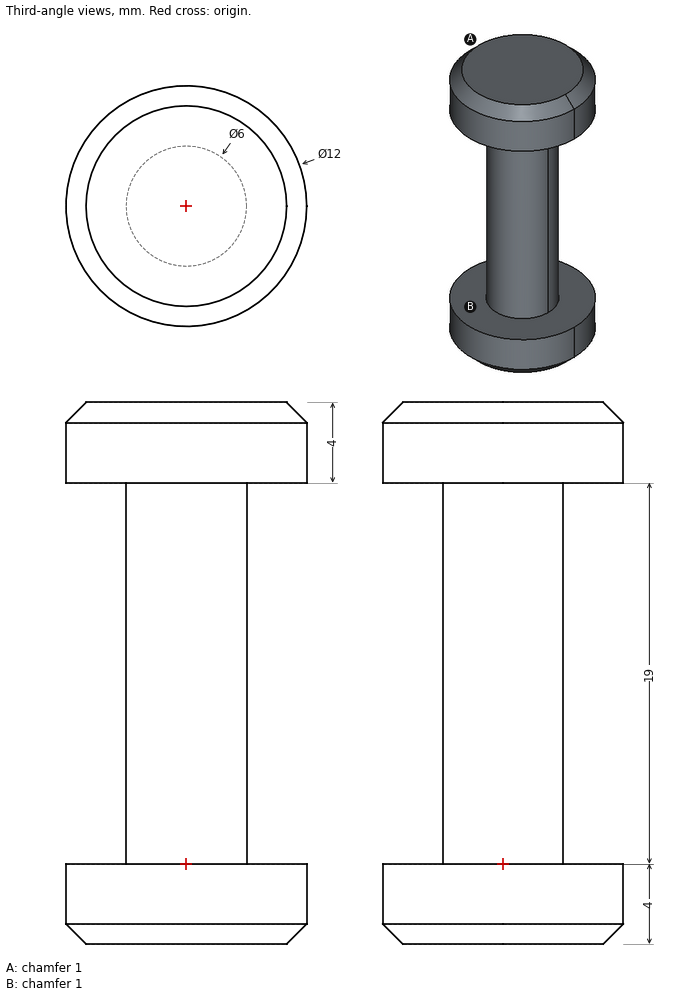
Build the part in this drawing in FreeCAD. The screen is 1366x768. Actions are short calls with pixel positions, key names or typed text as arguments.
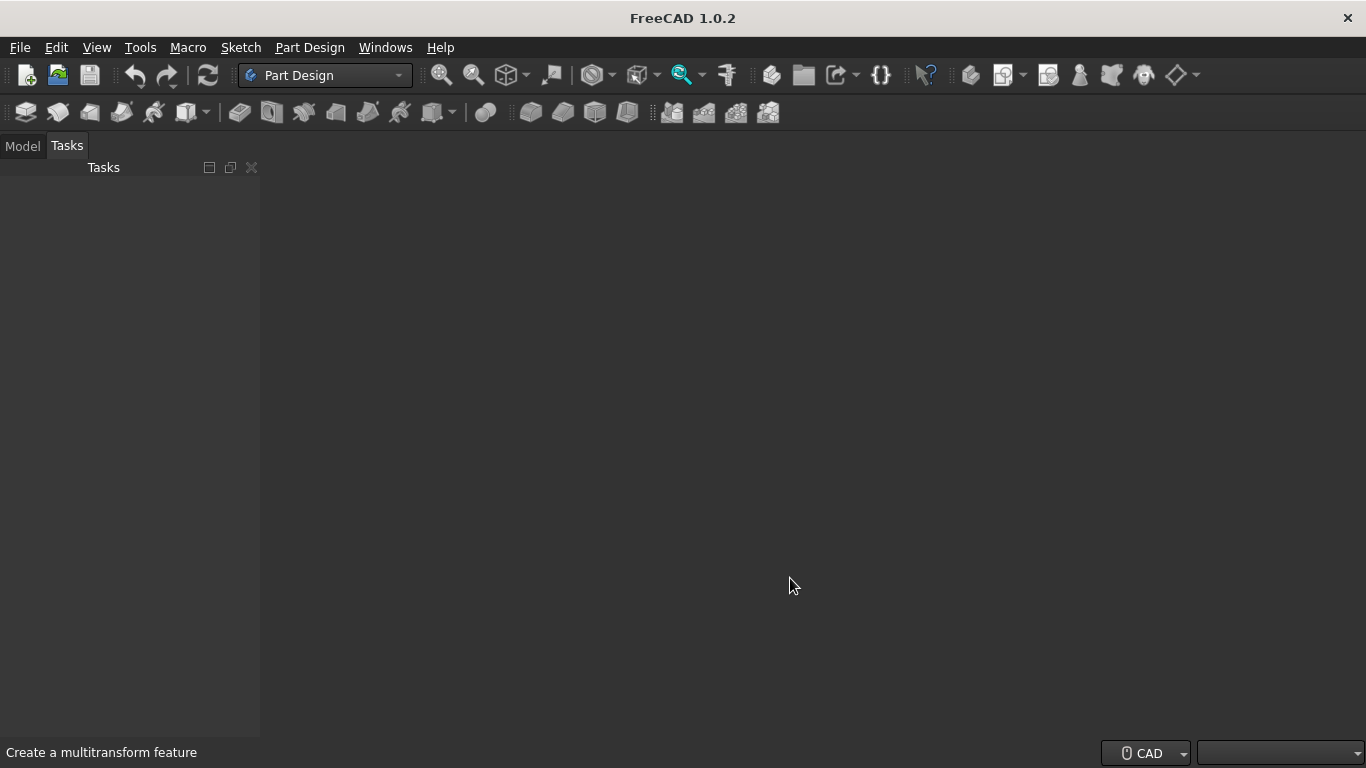
key(ctrl+n)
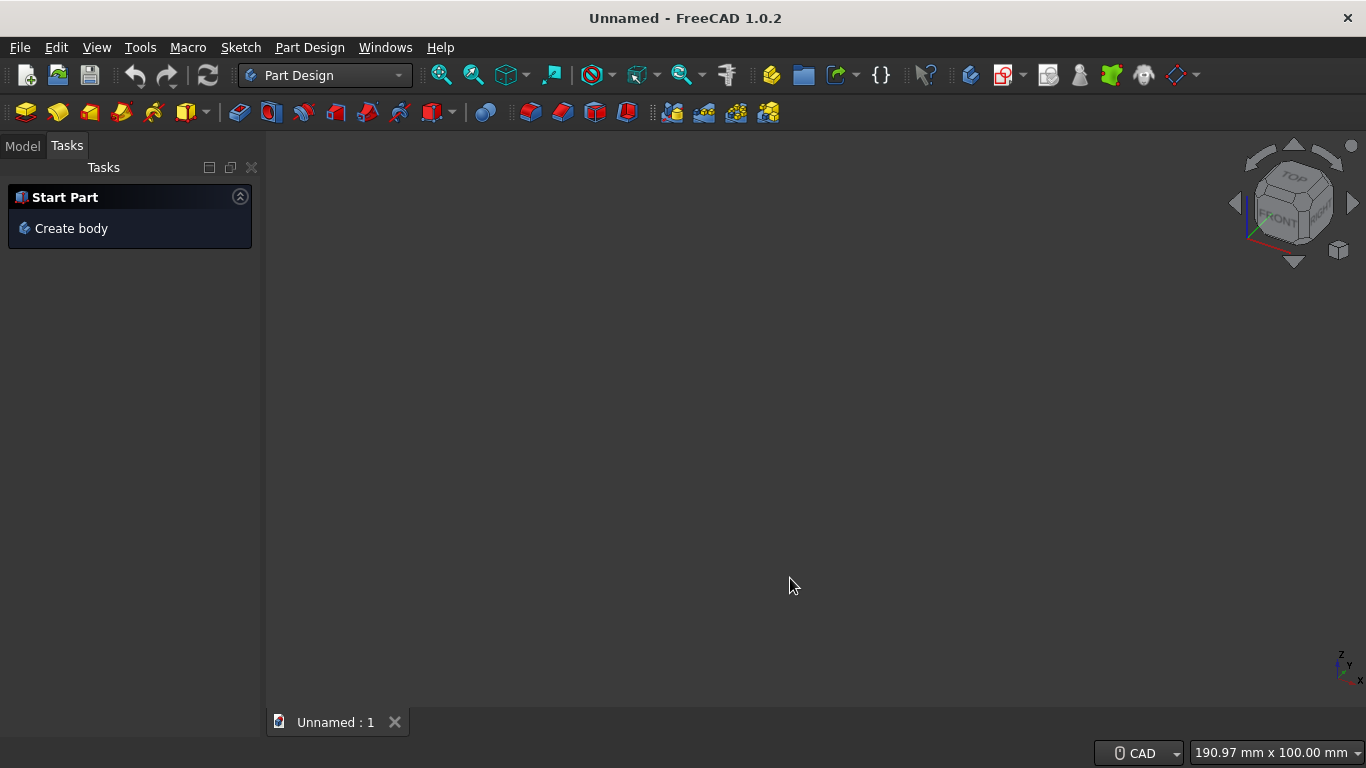
click(1004, 76)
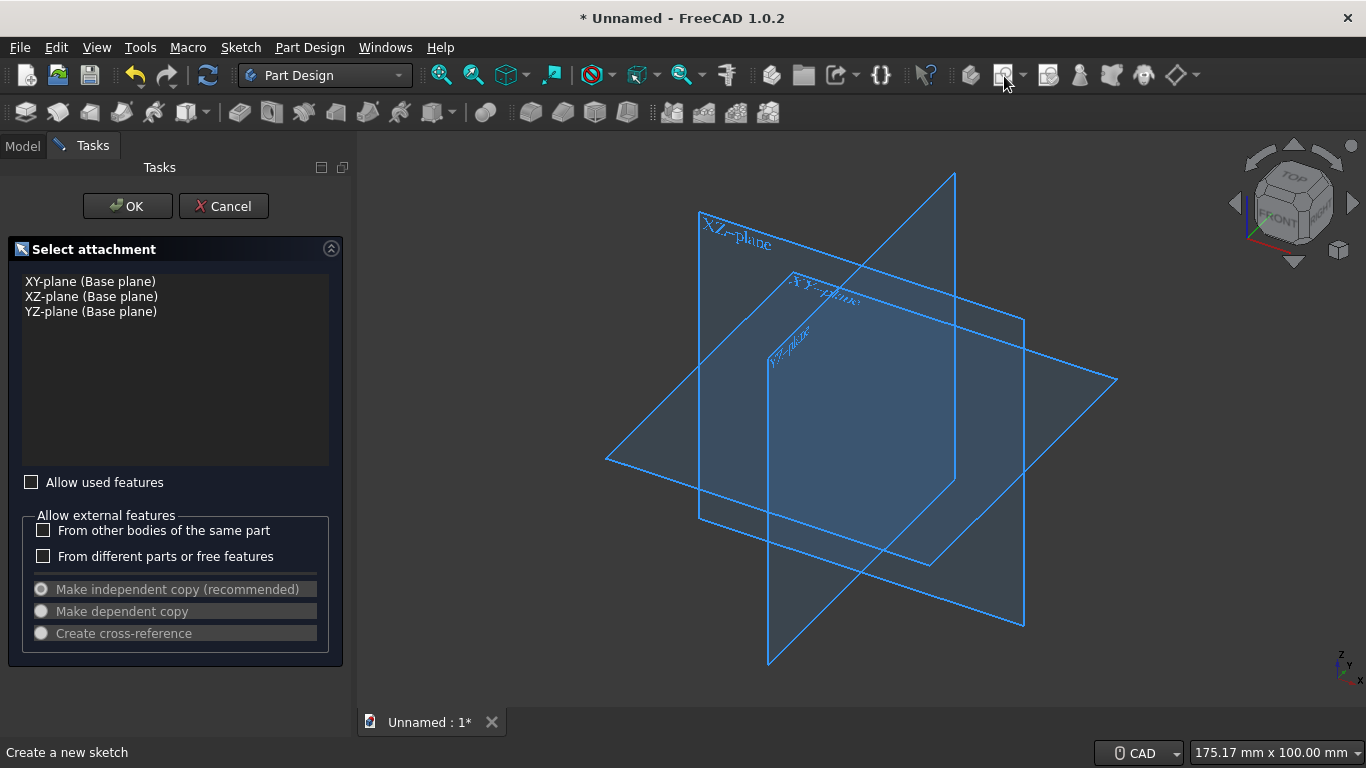
click(82, 282)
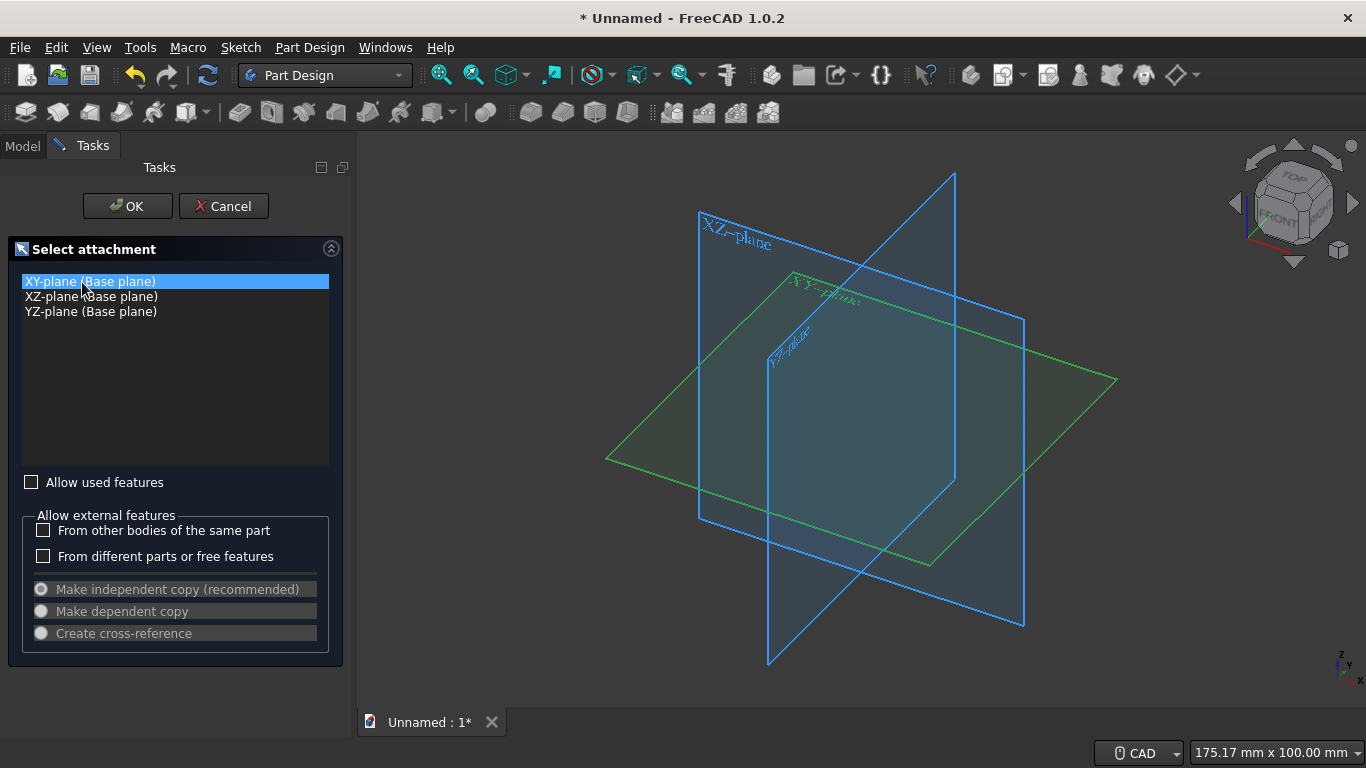
click(128, 206)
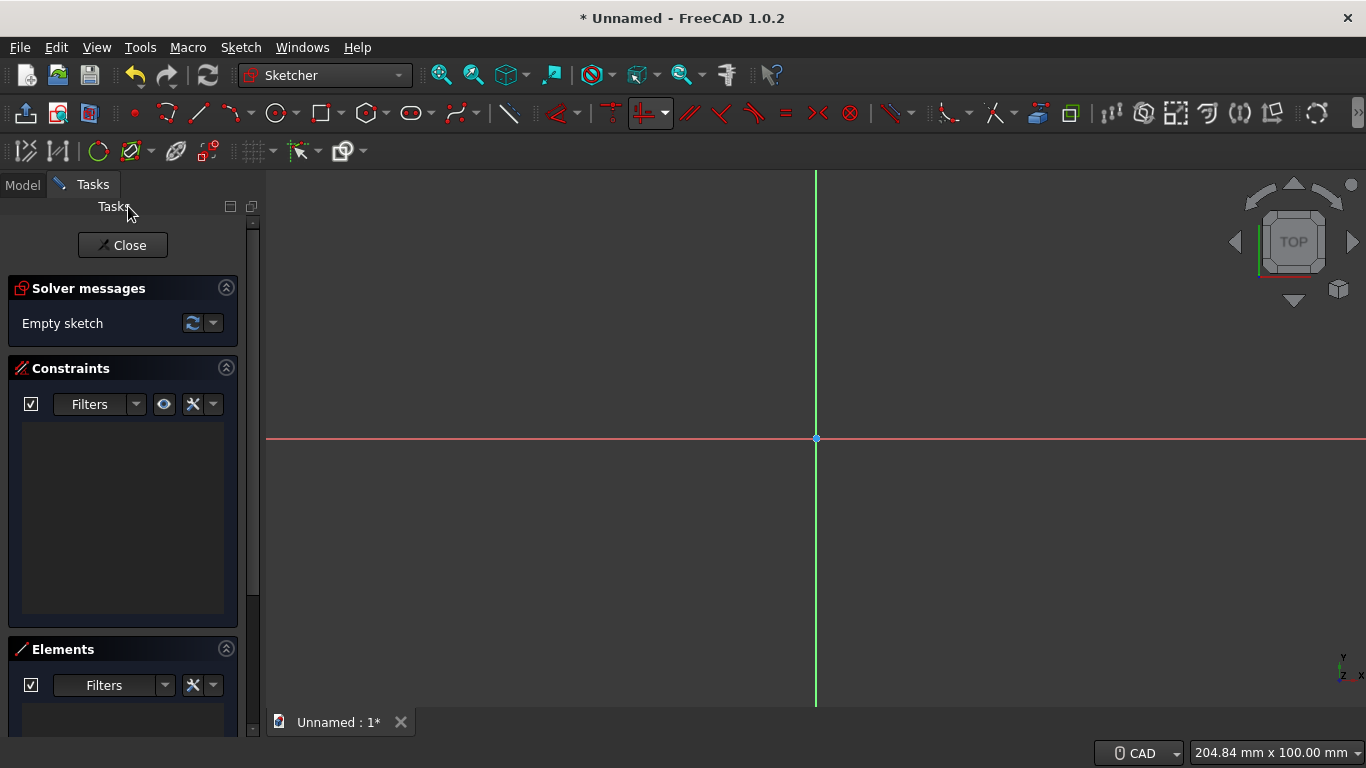
scroll(823, 438, up, 12)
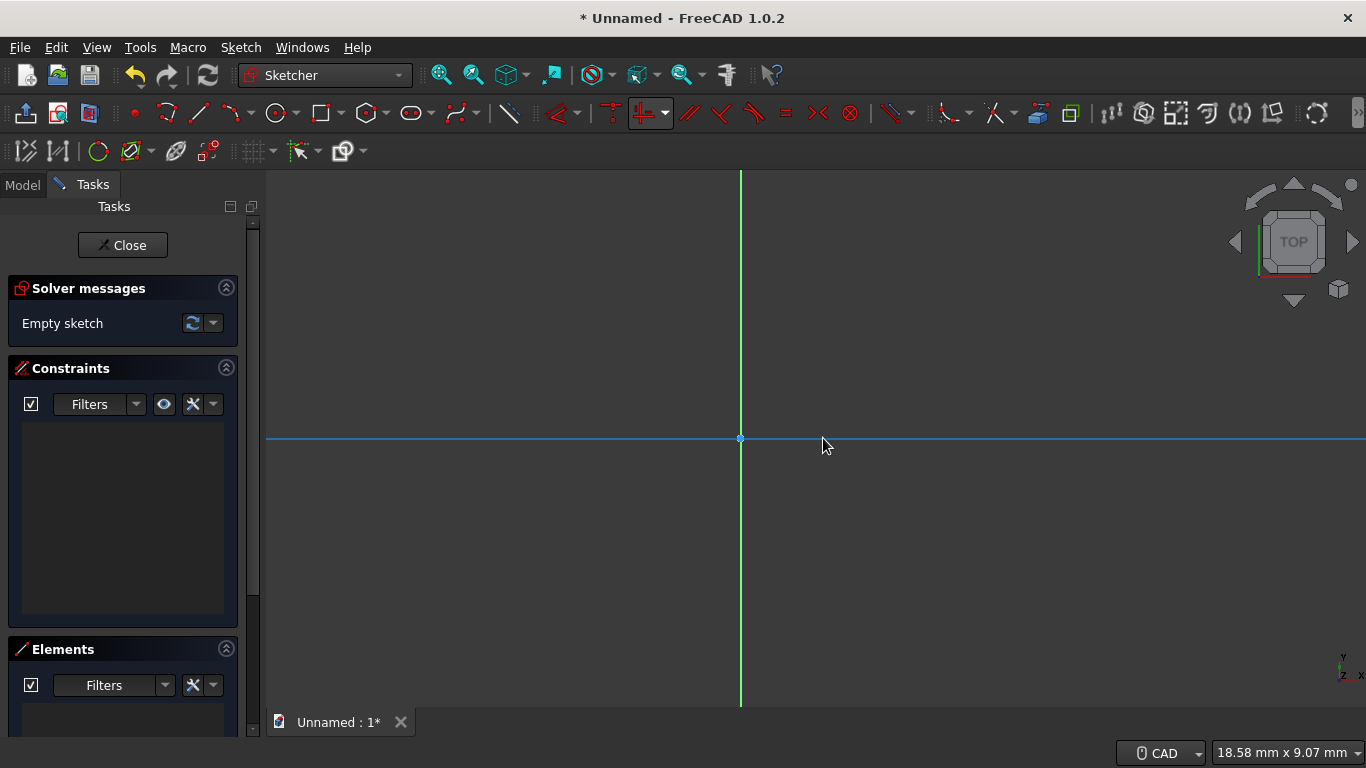
key(g)
key(c)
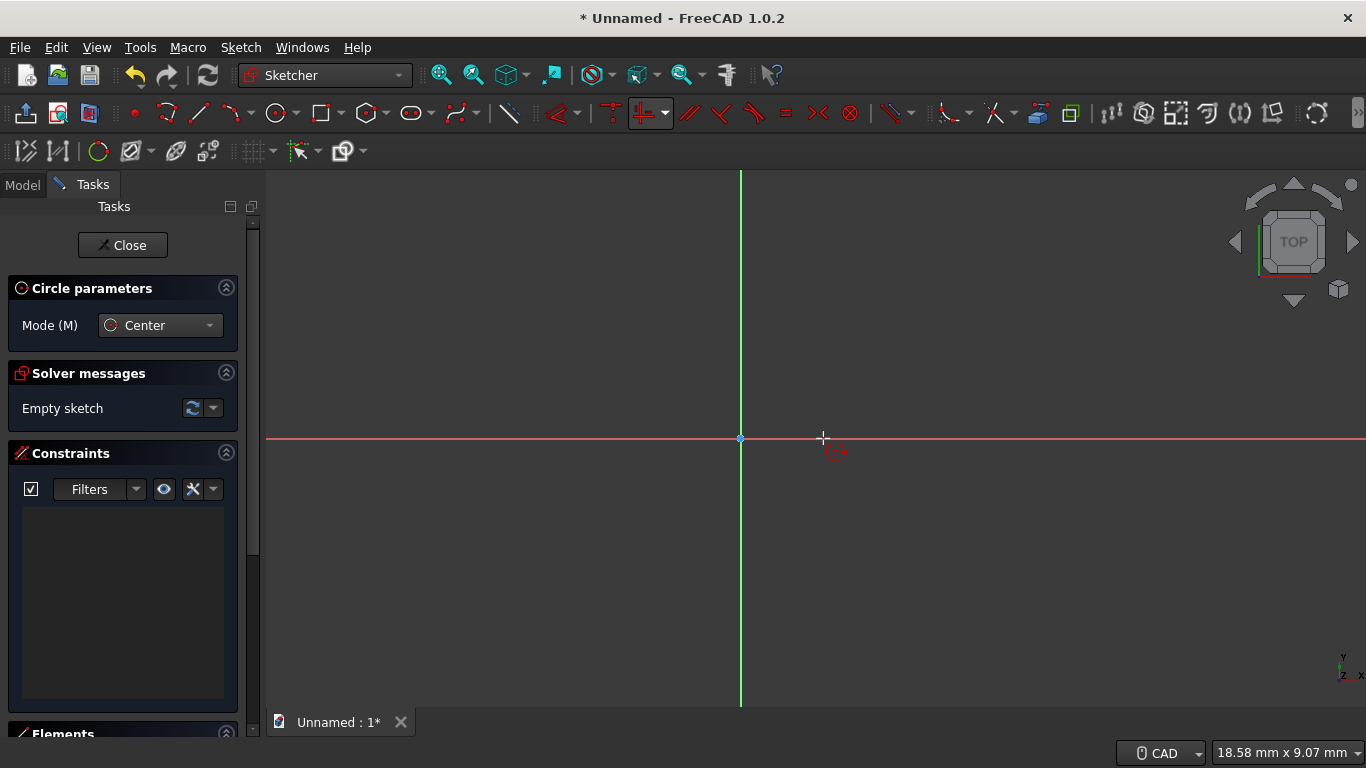
click(741, 438)
move(866, 313)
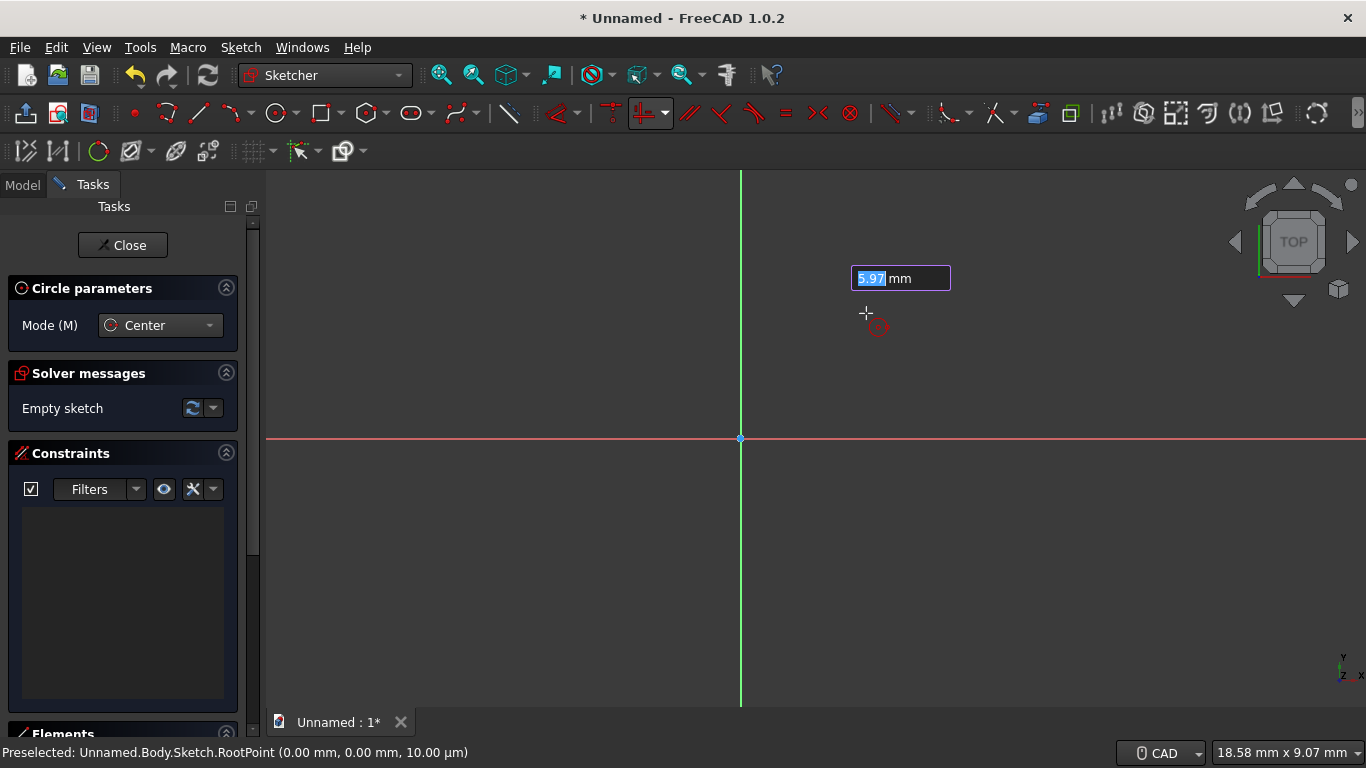
text(6)
key(Return)
key(Escape)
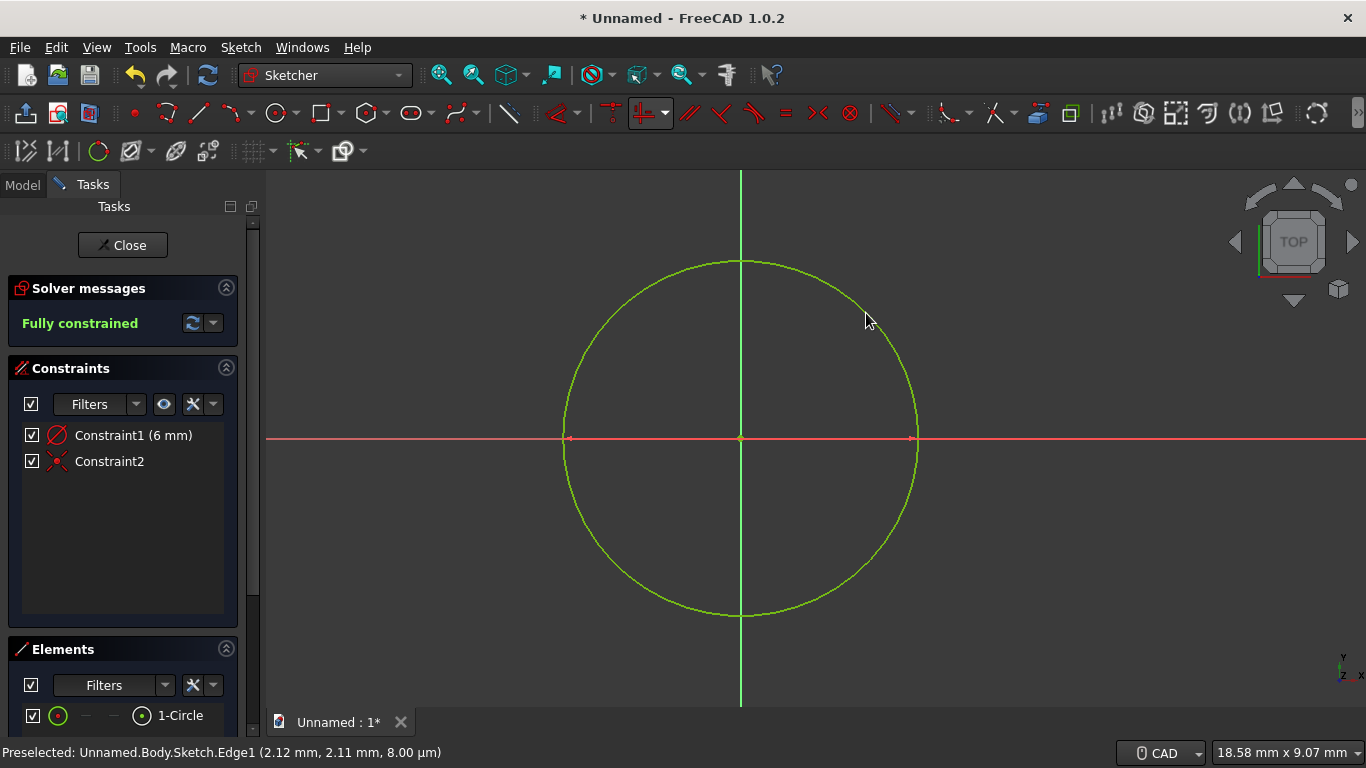
click(123, 245)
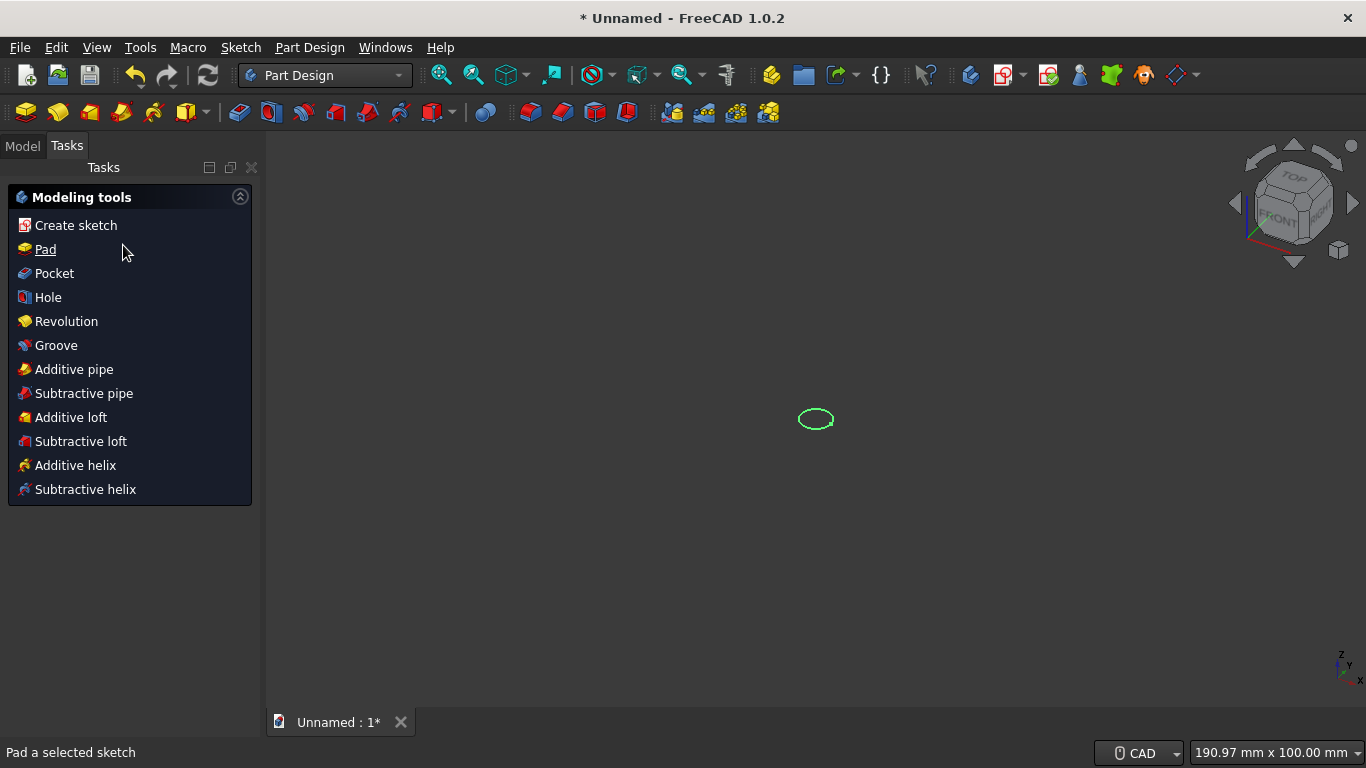
click(26, 112)